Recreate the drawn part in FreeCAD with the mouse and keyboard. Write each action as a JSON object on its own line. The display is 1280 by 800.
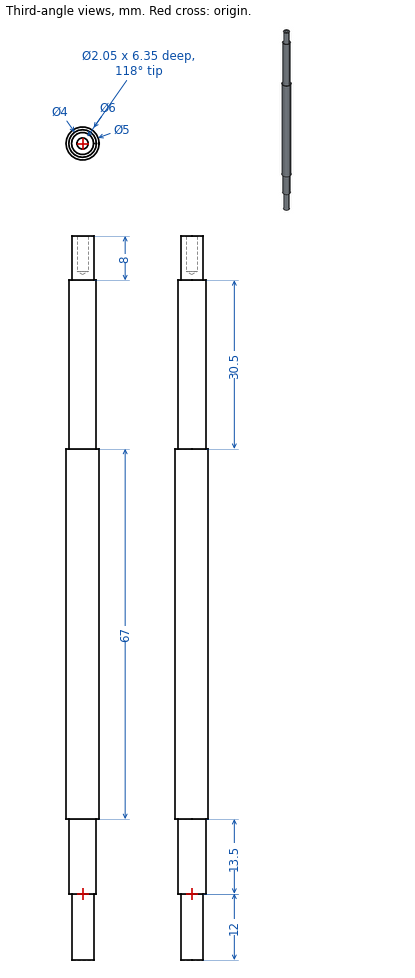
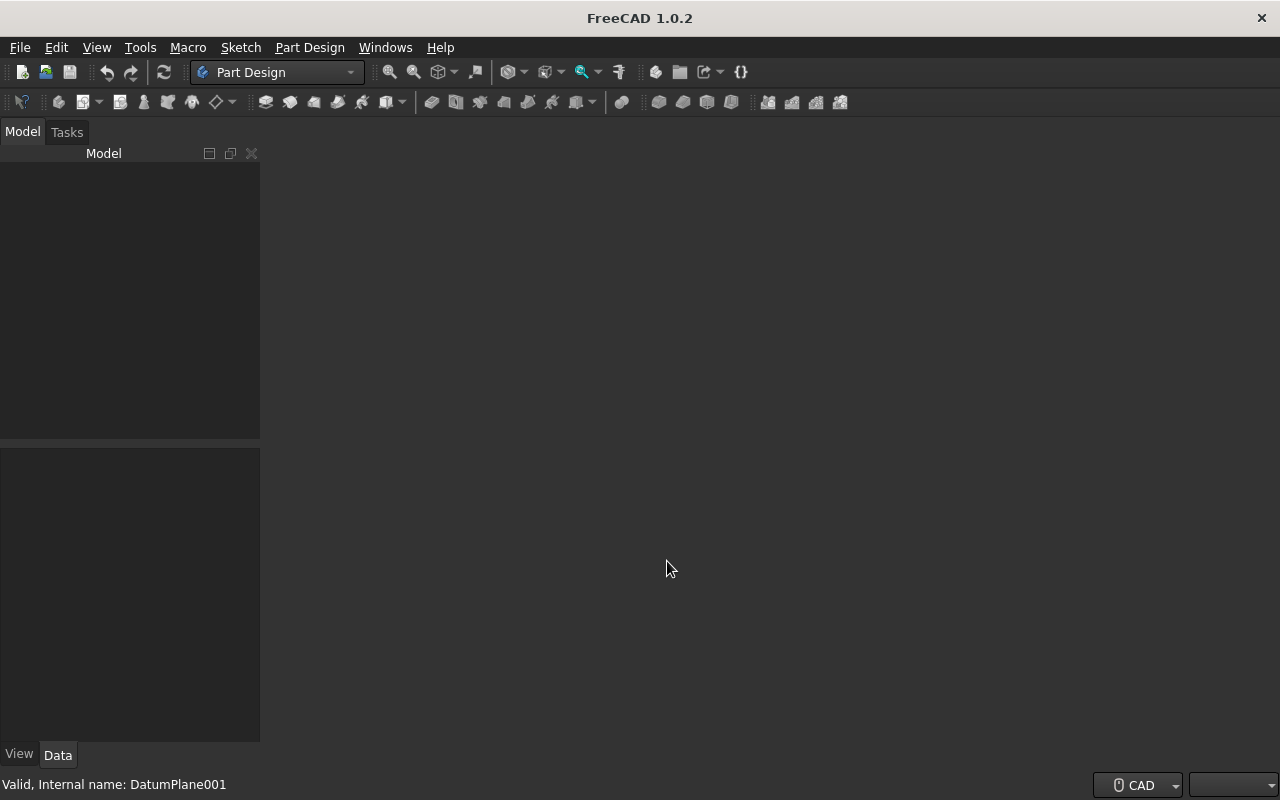
{"action": "left_click", "coordinate": [22, 72]}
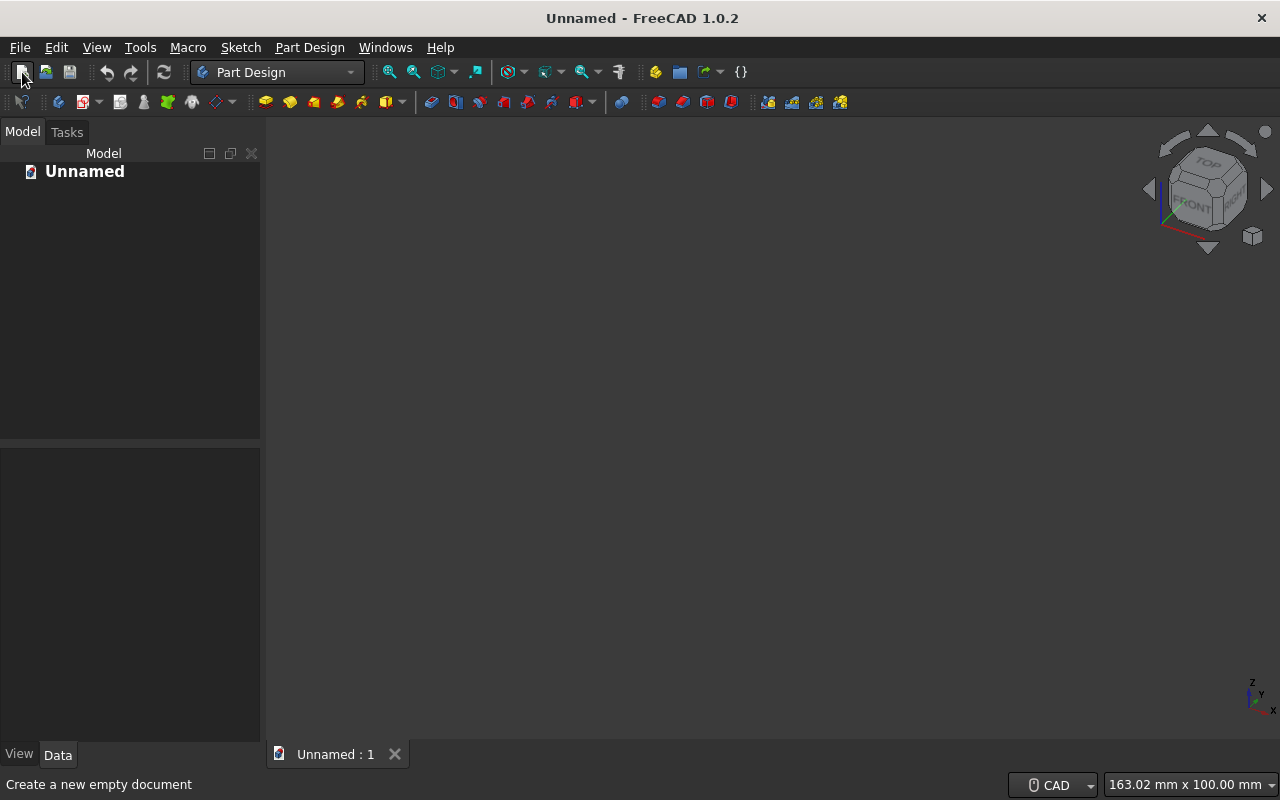
{"action": "left_click", "coordinate": [84, 102]}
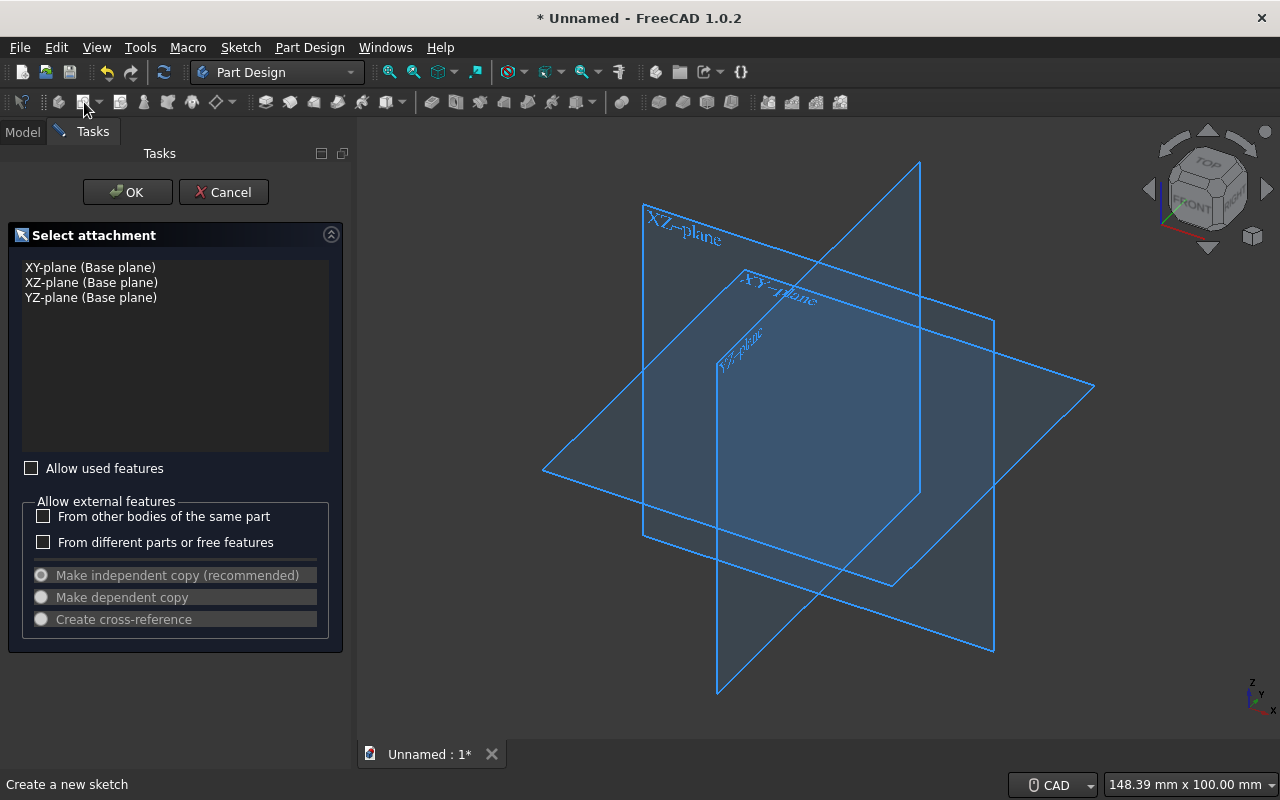
{"action": "left_click", "coordinate": [82, 268]}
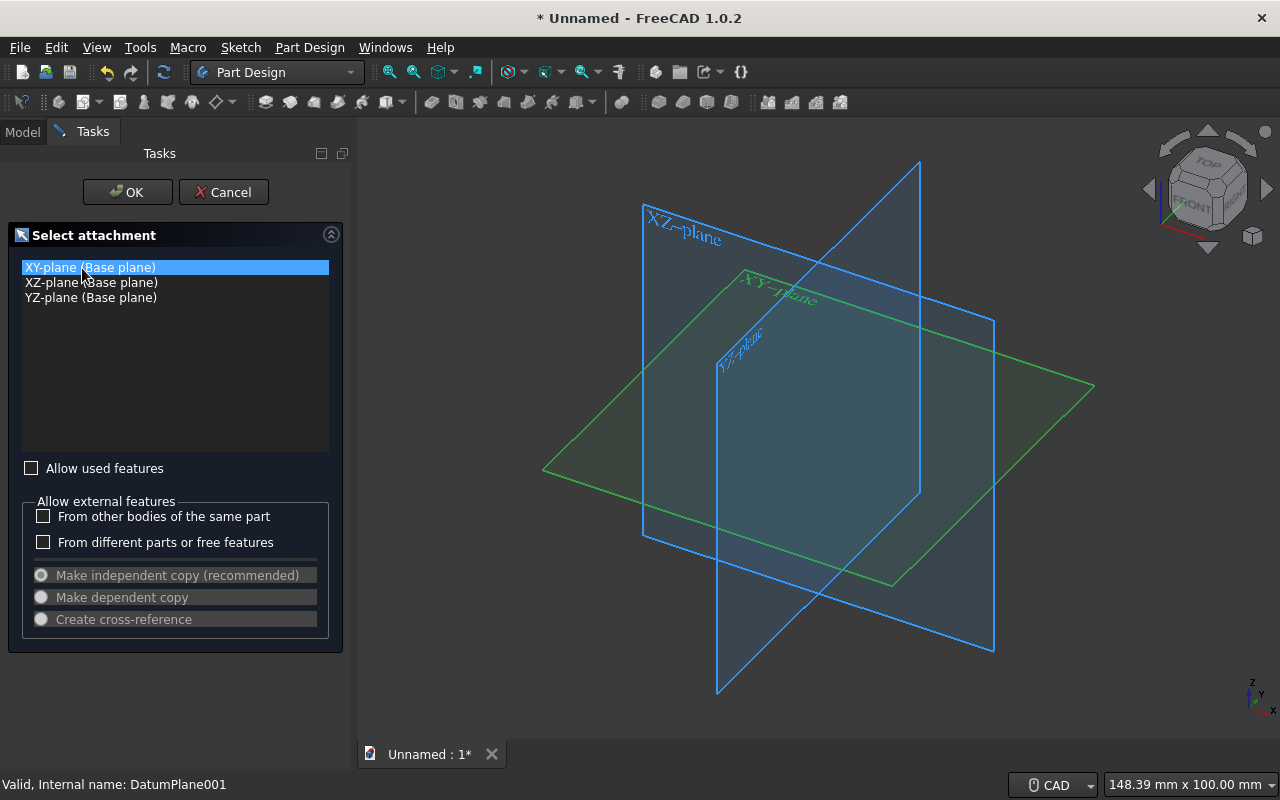
{"action": "left_click", "coordinate": [128, 192]}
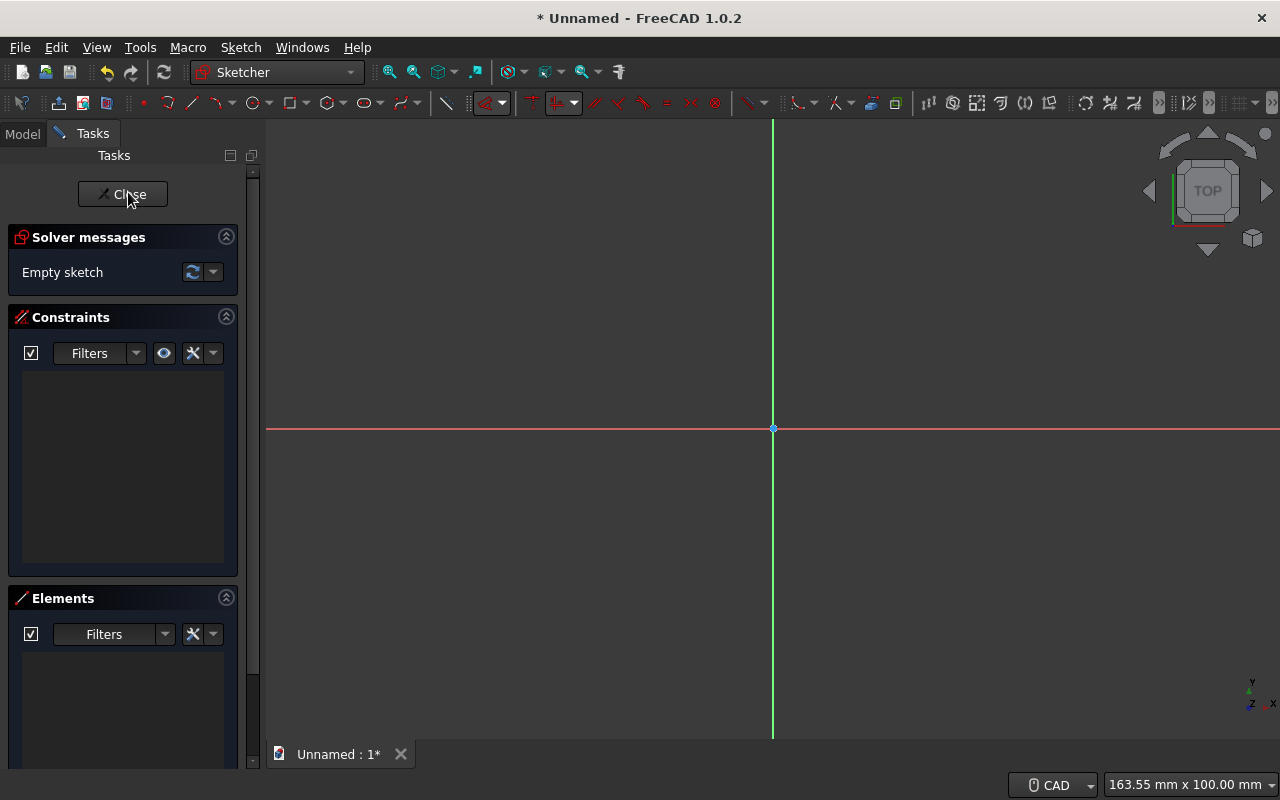
{"action": "scroll", "coordinate": [778, 429], "scroll_direction": "up", "scroll_amount": 13}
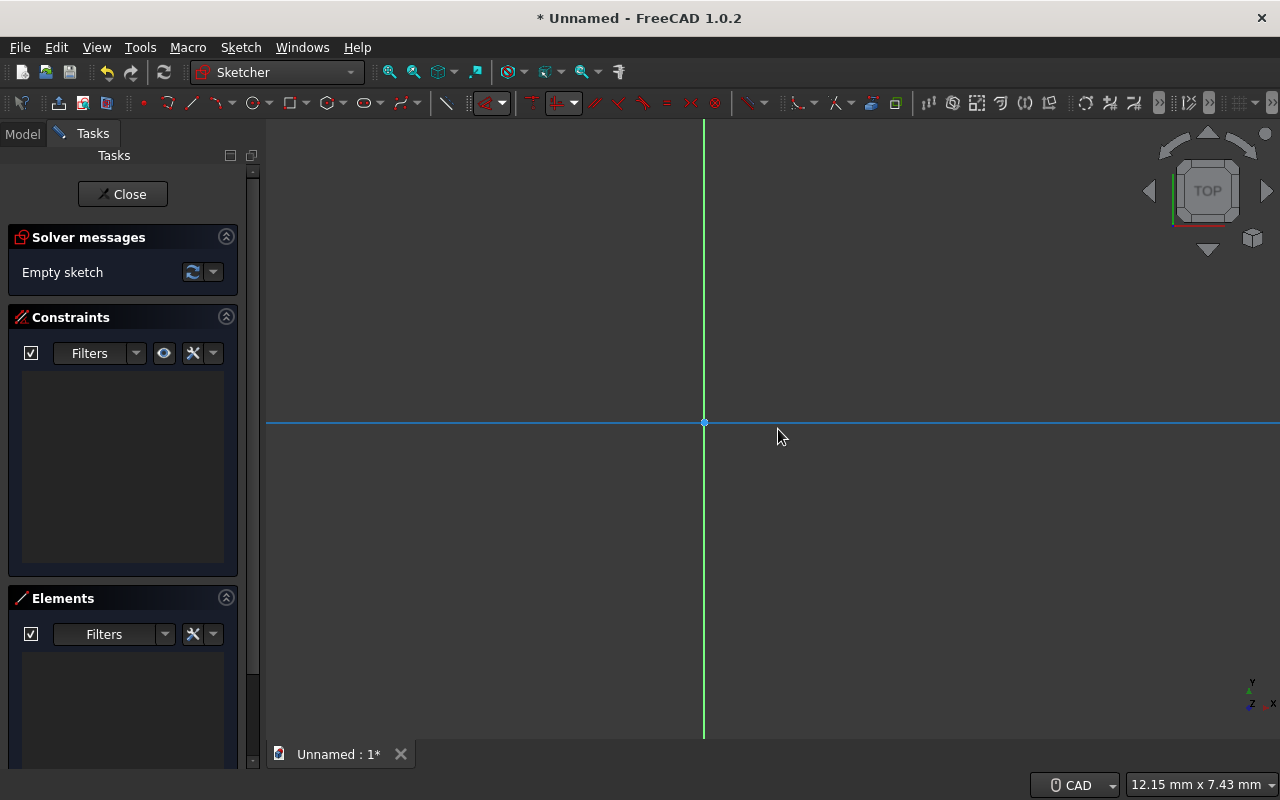
{"action": "left_click", "coordinate": [254, 104]}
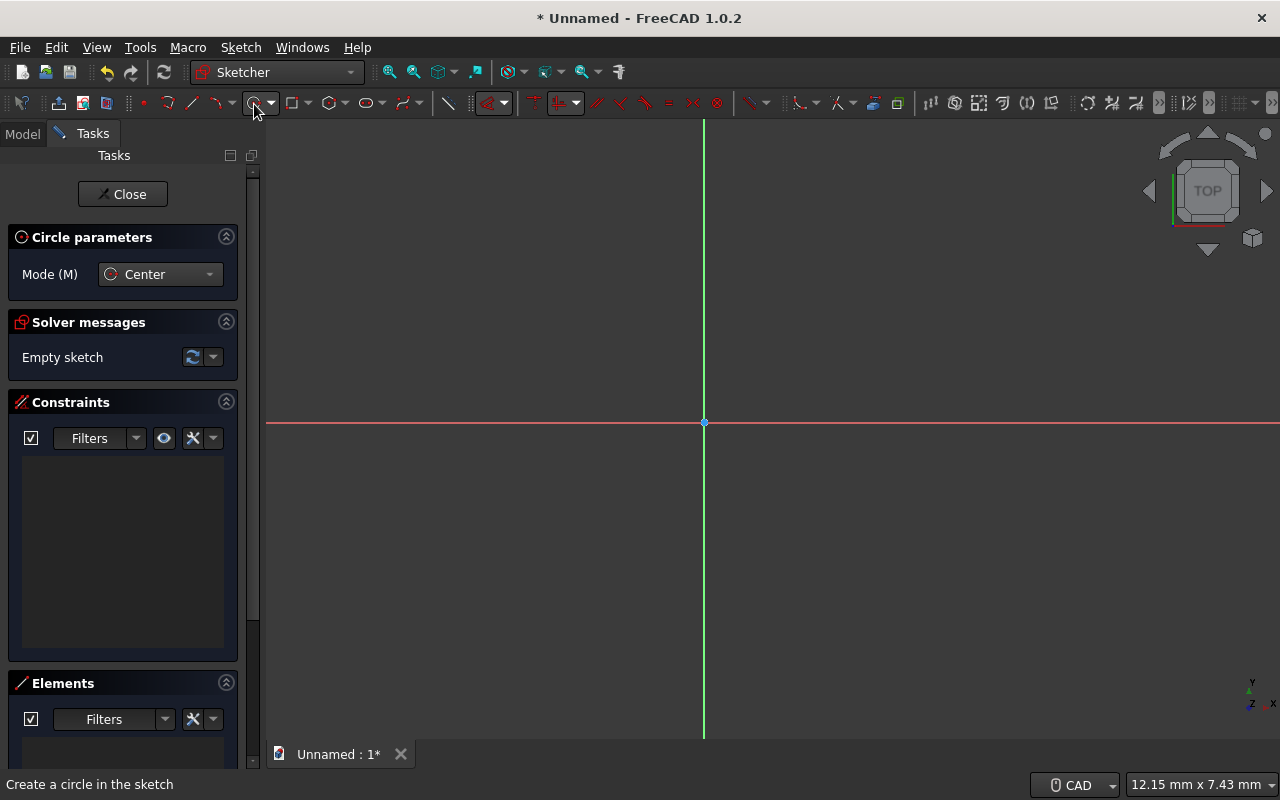
{"action": "left_click", "coordinate": [704, 423]}
{"action": "left_click", "coordinate": [852, 275]}
{"action": "key", "text": "Escape"}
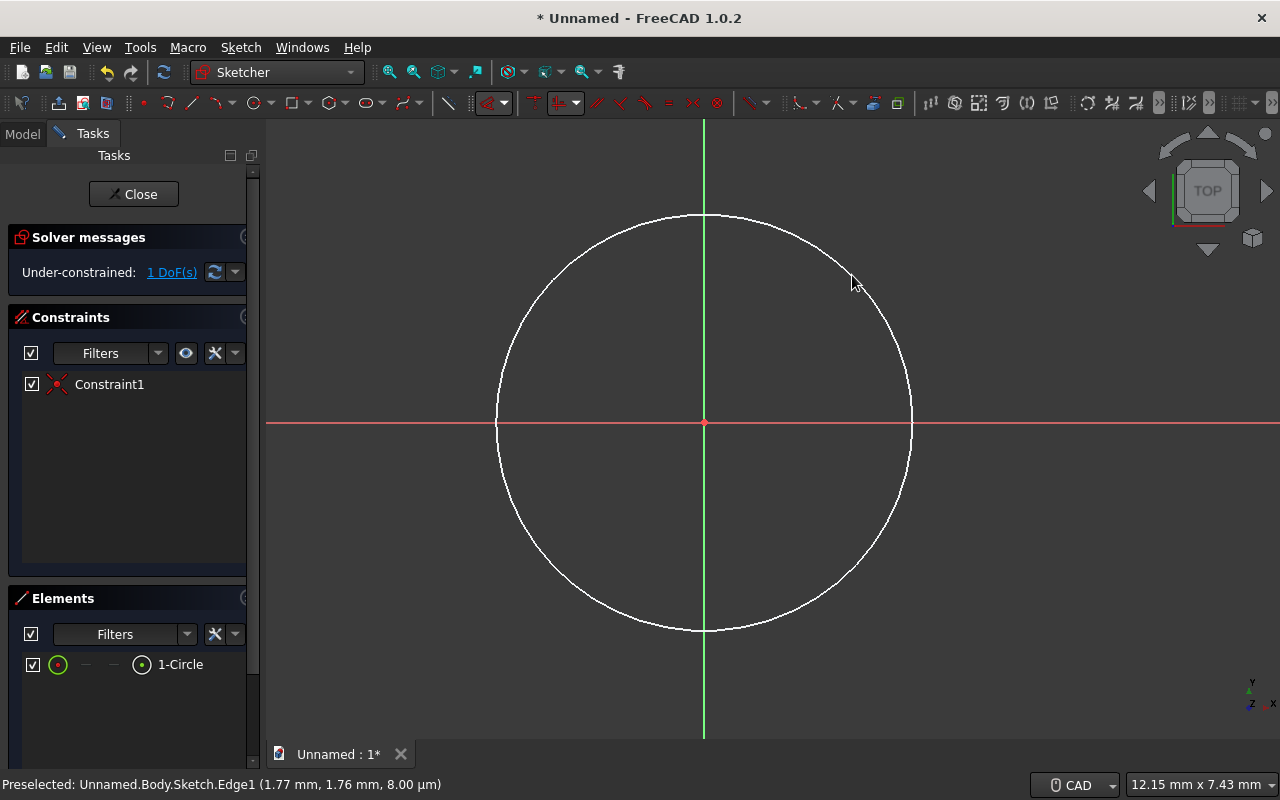
{"action": "left_click", "coordinate": [488, 104]}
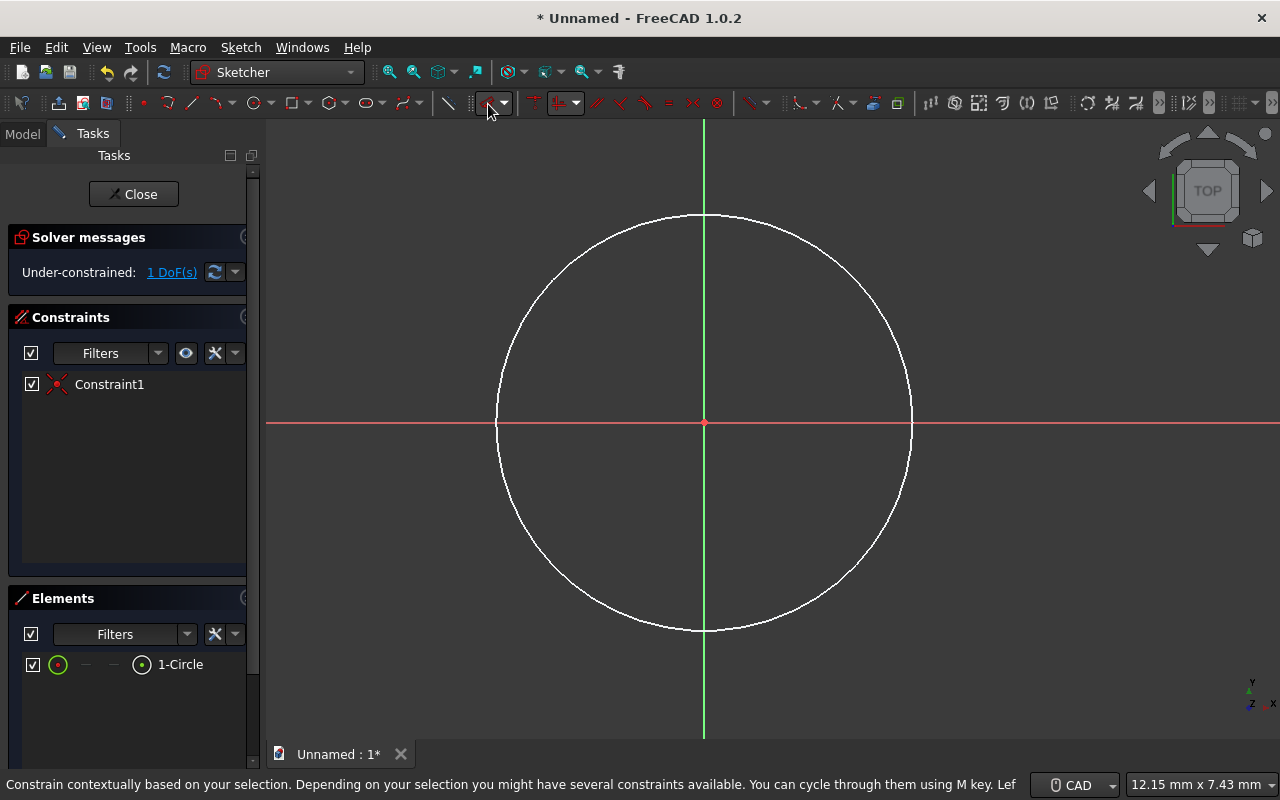
{"action": "left_click", "coordinate": [851, 275]}
{"action": "left_click", "coordinate": [874, 252]}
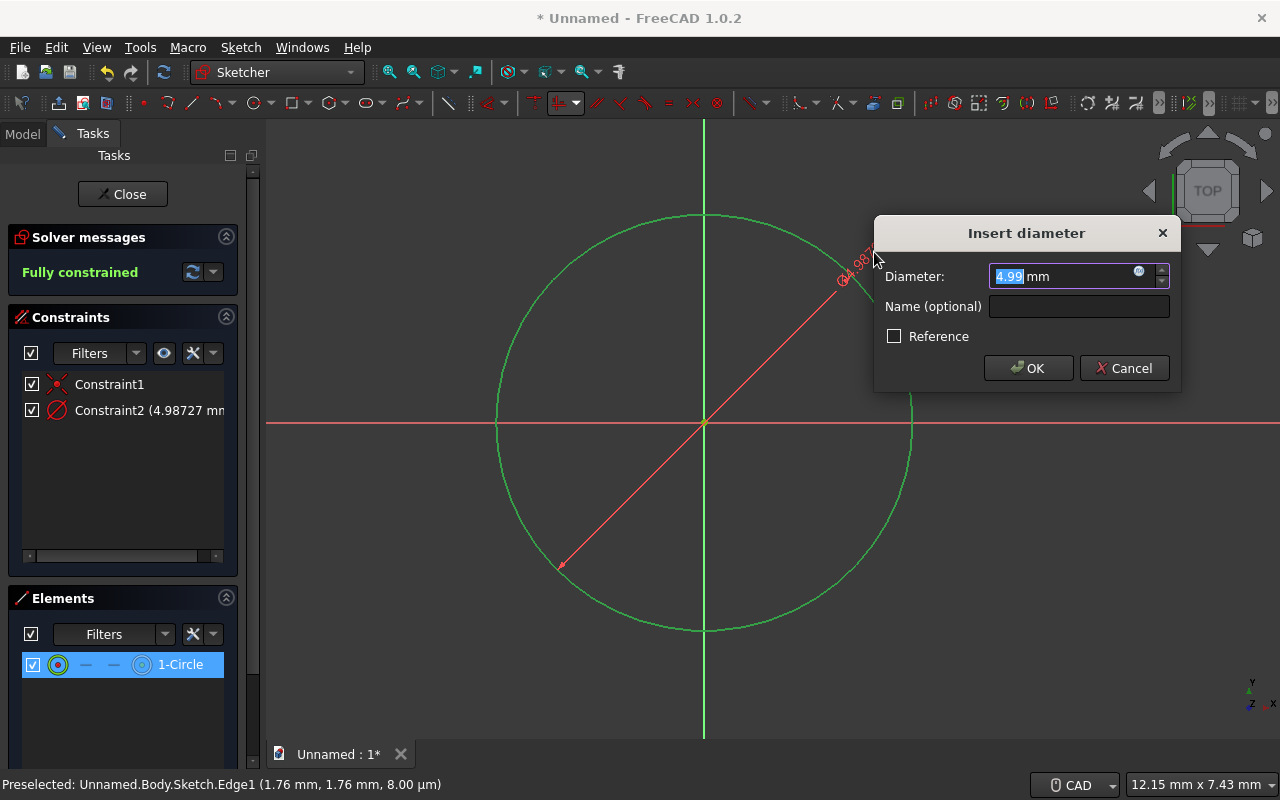
{"action": "type", "text": "5"}
{"action": "key", "text": "Return"}
{"action": "key", "text": "Escape"}